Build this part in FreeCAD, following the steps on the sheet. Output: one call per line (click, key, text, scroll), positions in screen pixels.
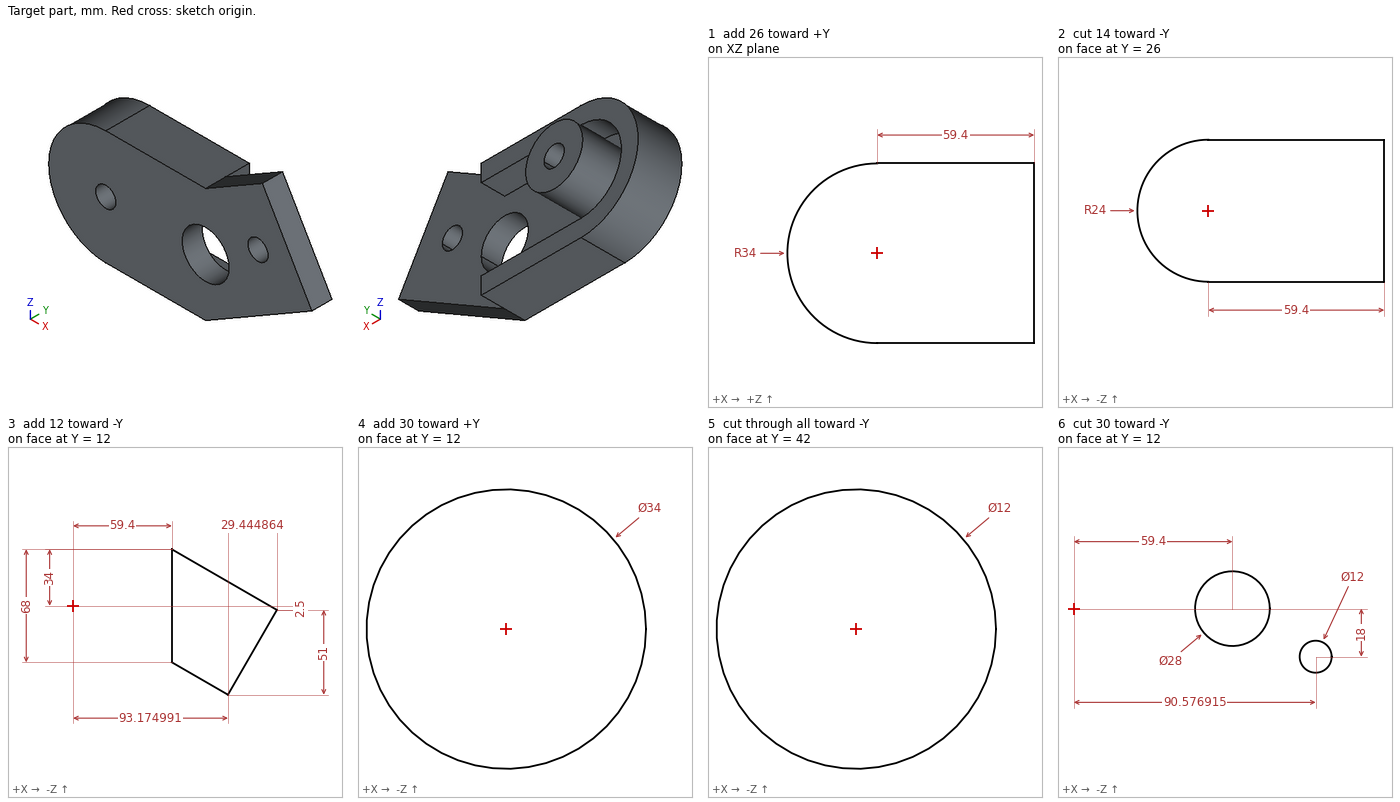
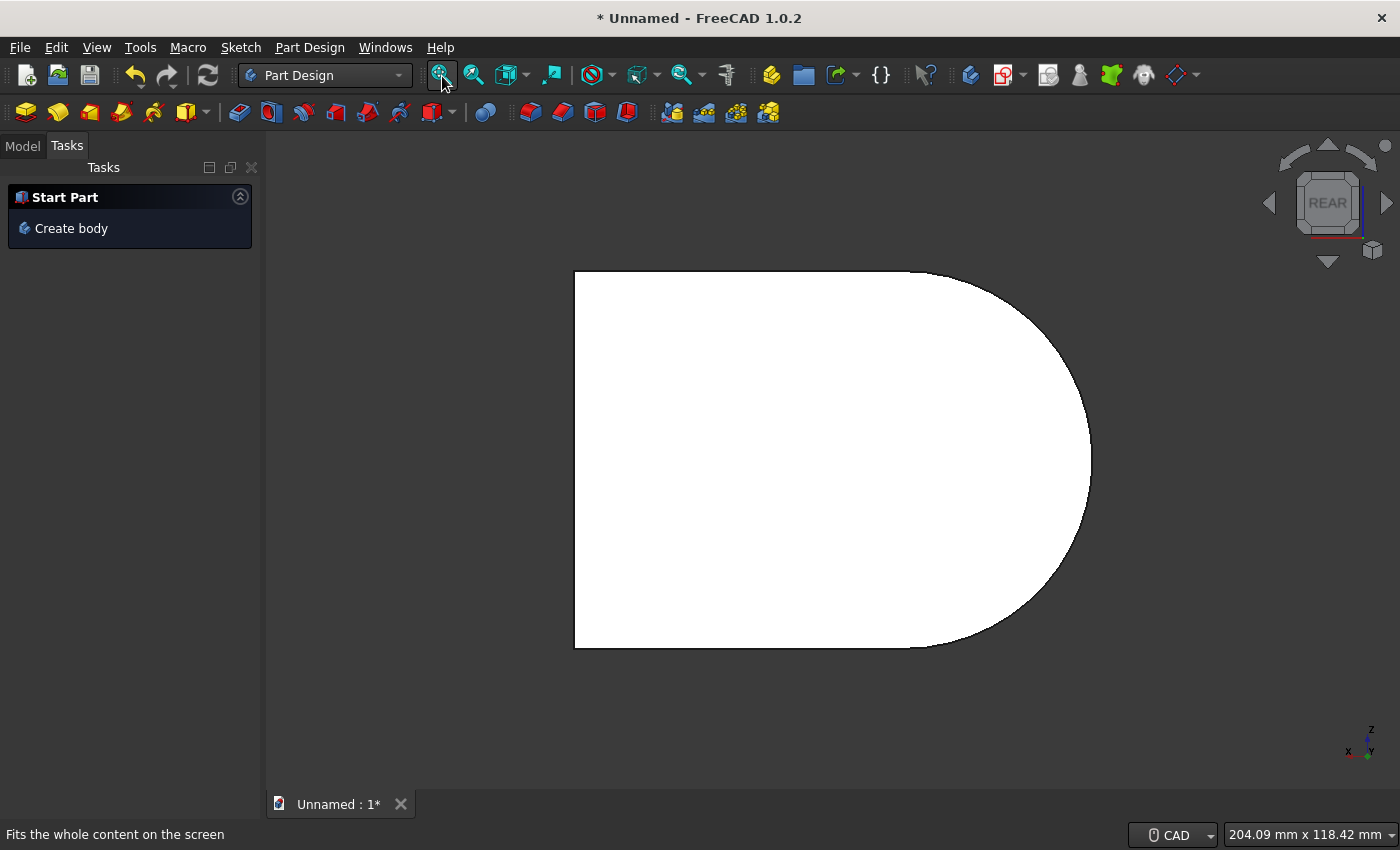
click(833, 459)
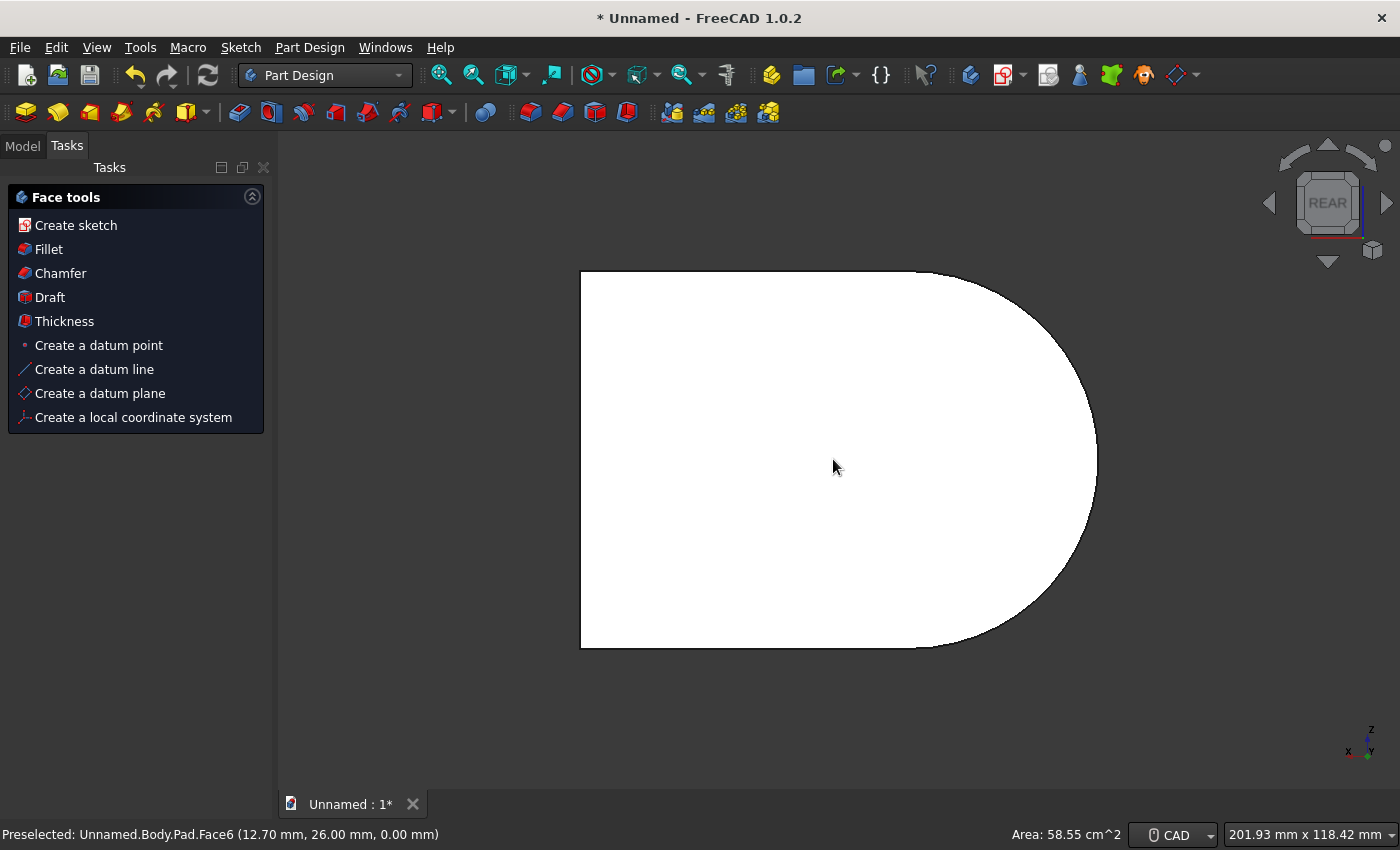
click(1004, 76)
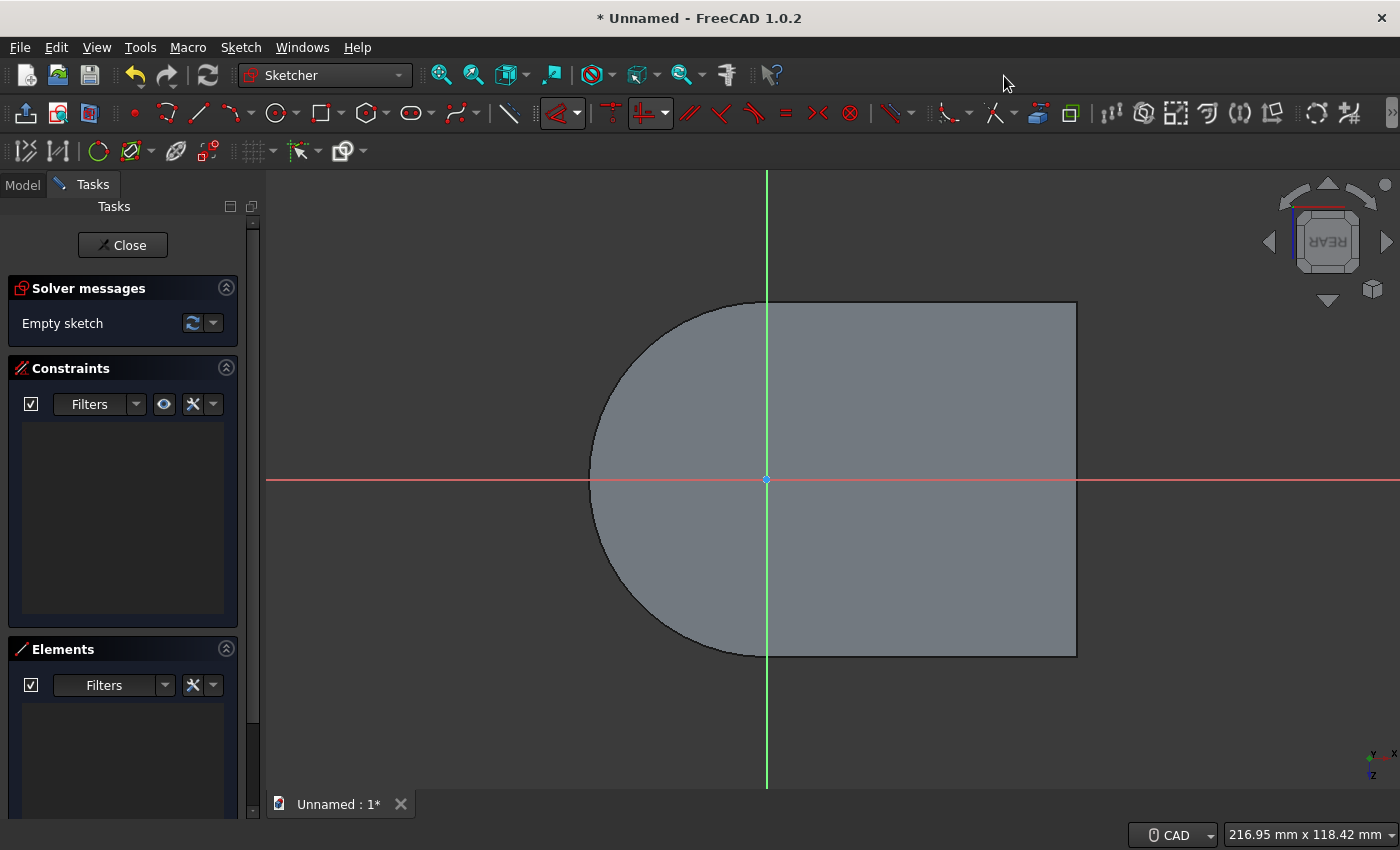
scroll(1052, 480, up, 2)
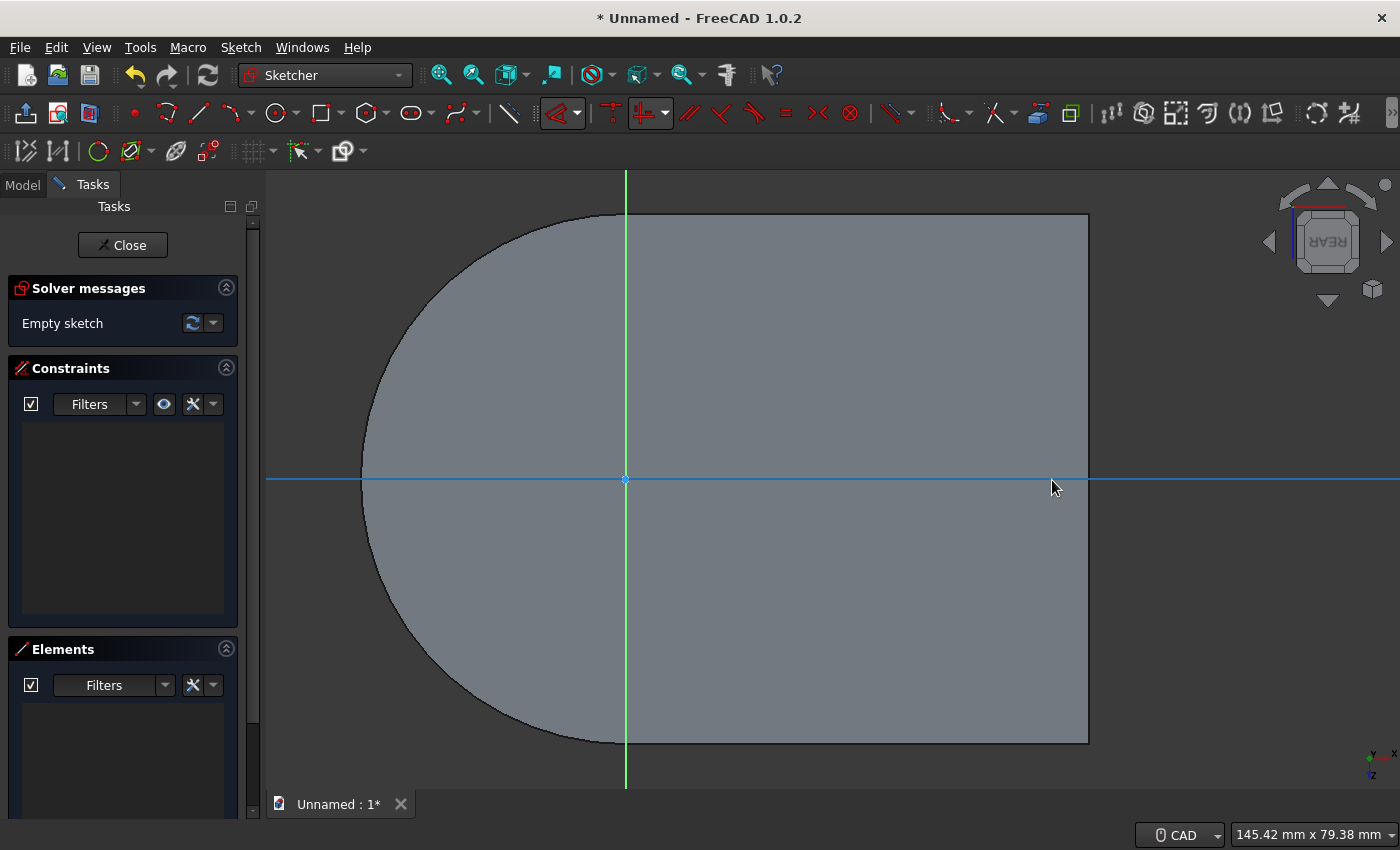
click(168, 114)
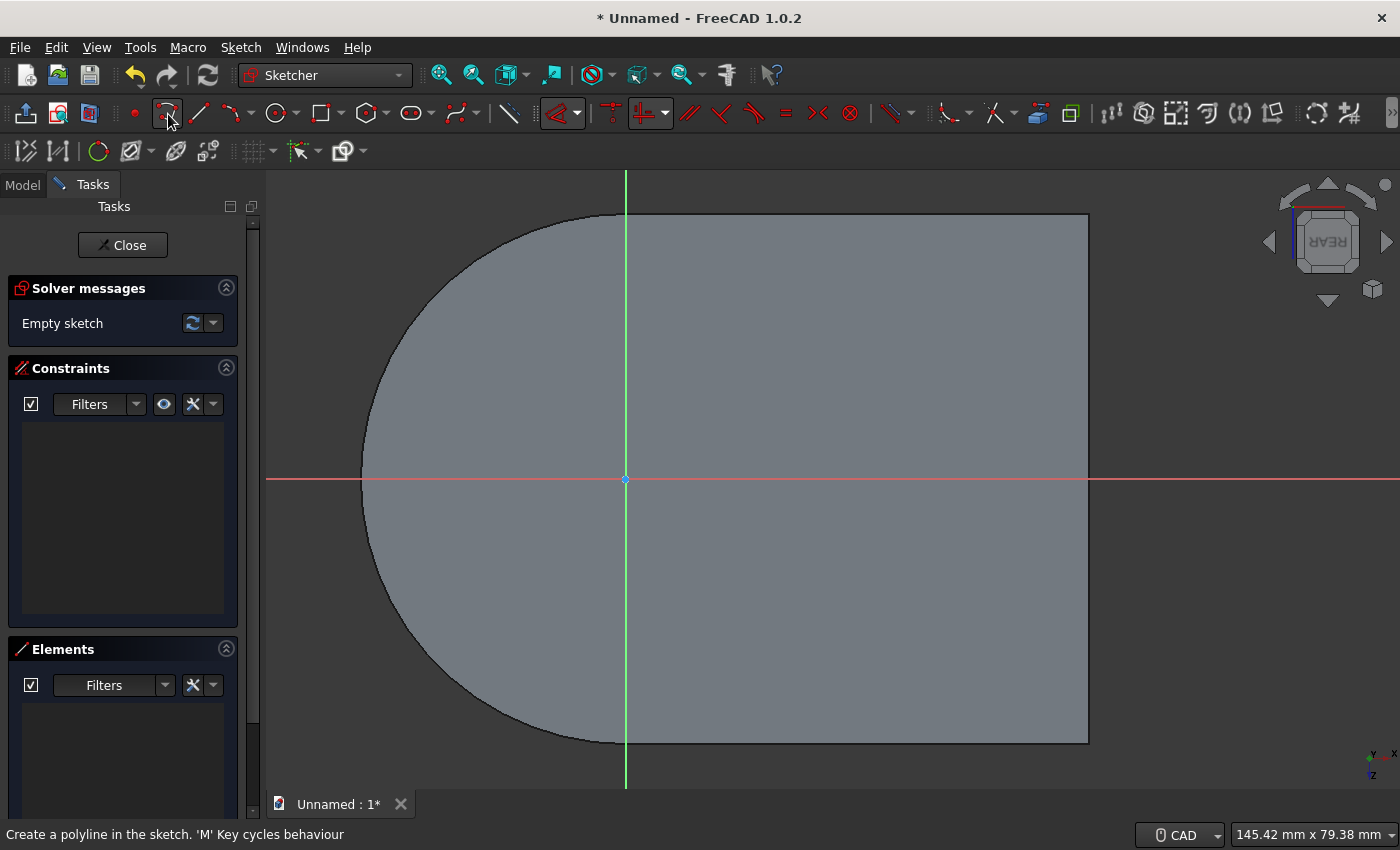
click(626, 666)
click(1089, 666)
click(1089, 292)
click(626, 292)
right_click(626, 292)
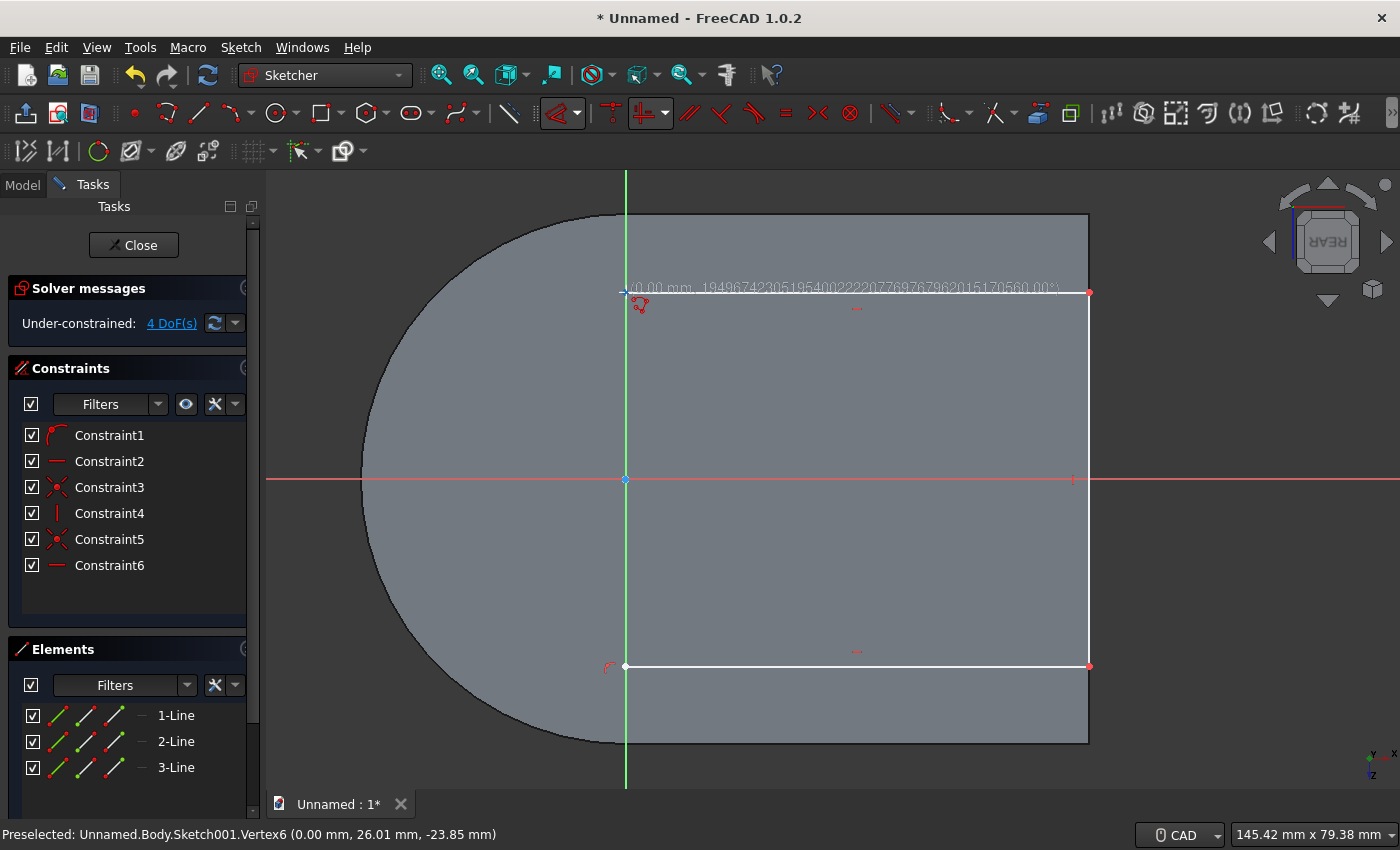
click(232, 114)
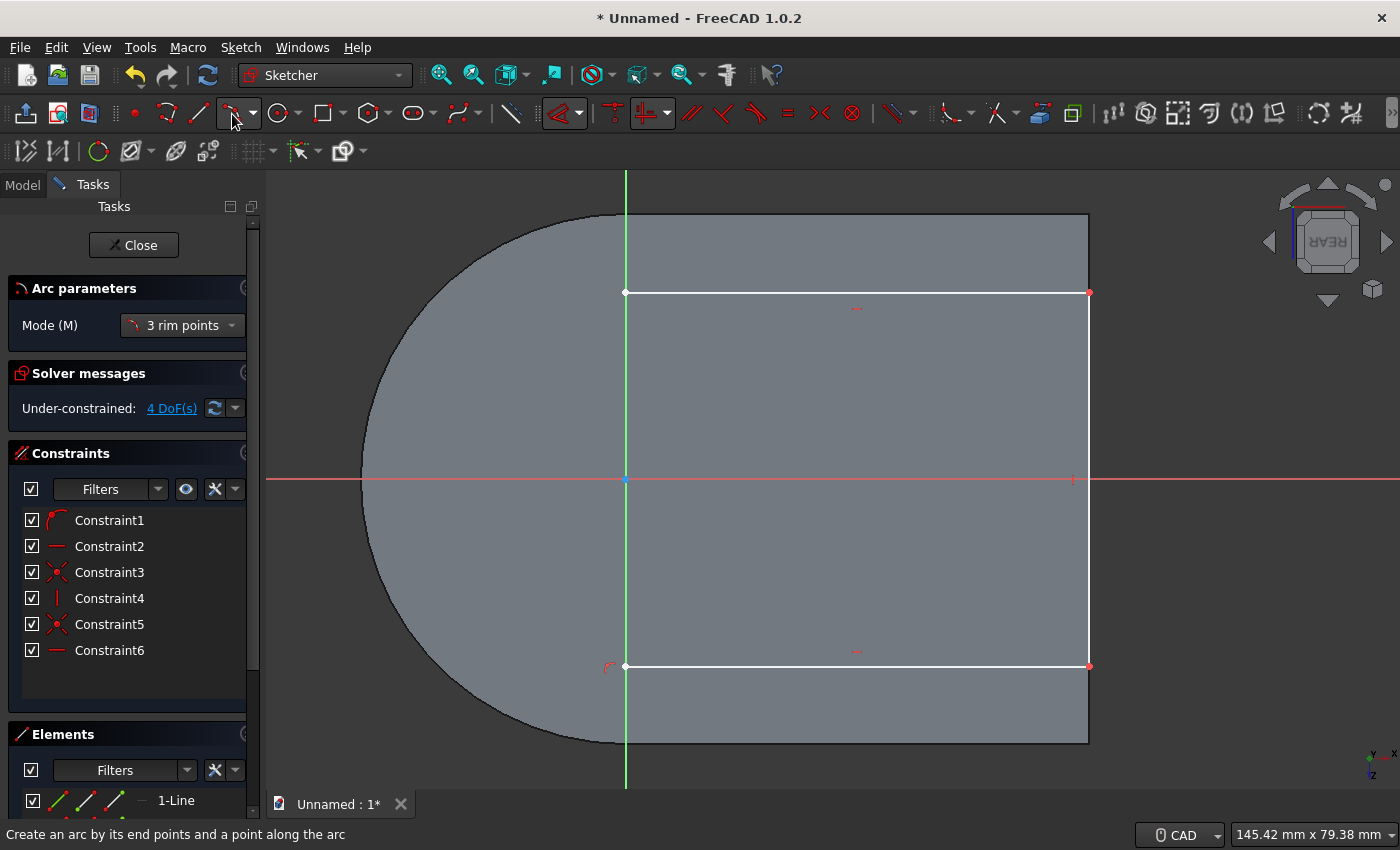
click(626, 293)
click(626, 667)
click(448, 421)
key(Escape)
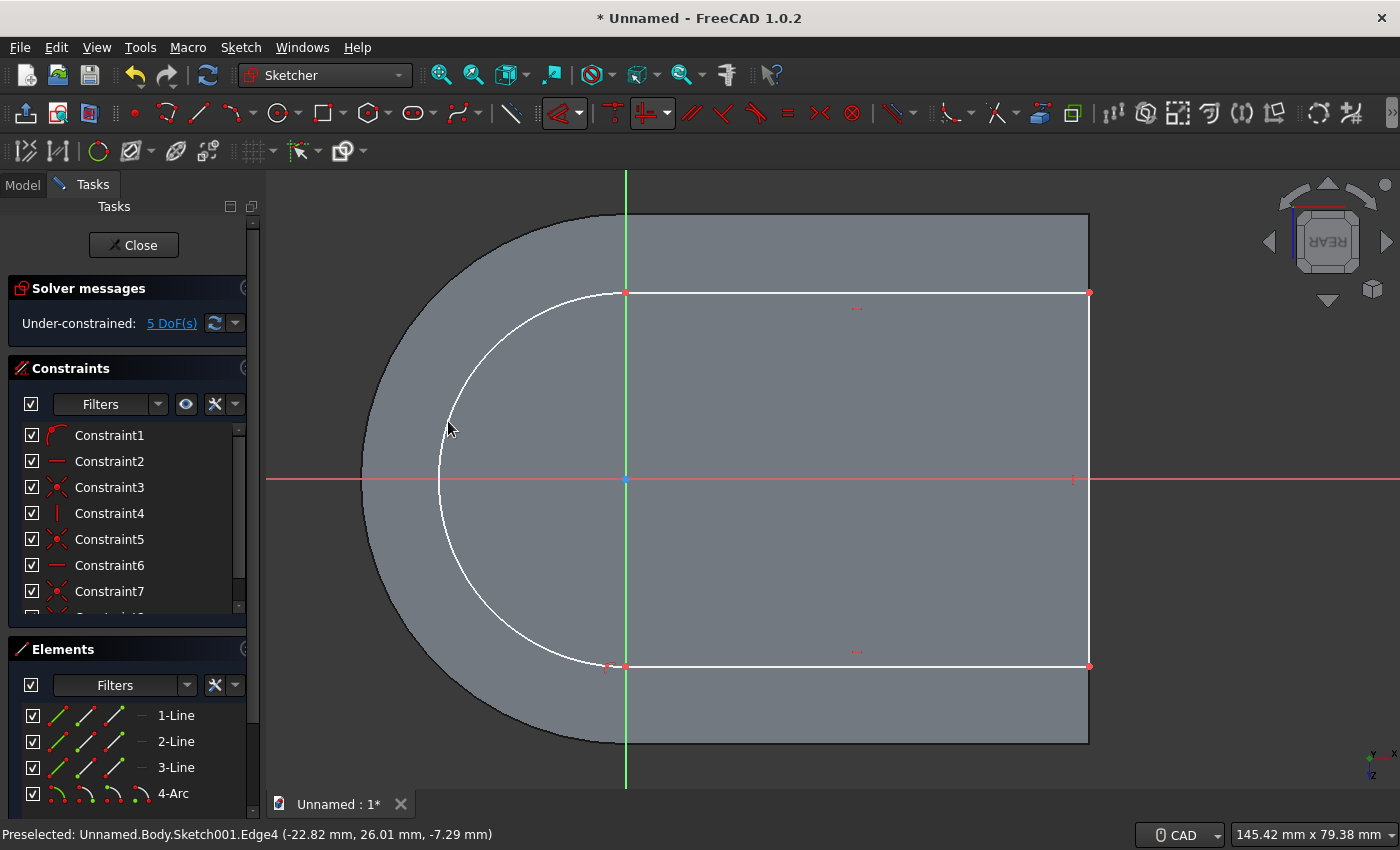
click(765, 667)